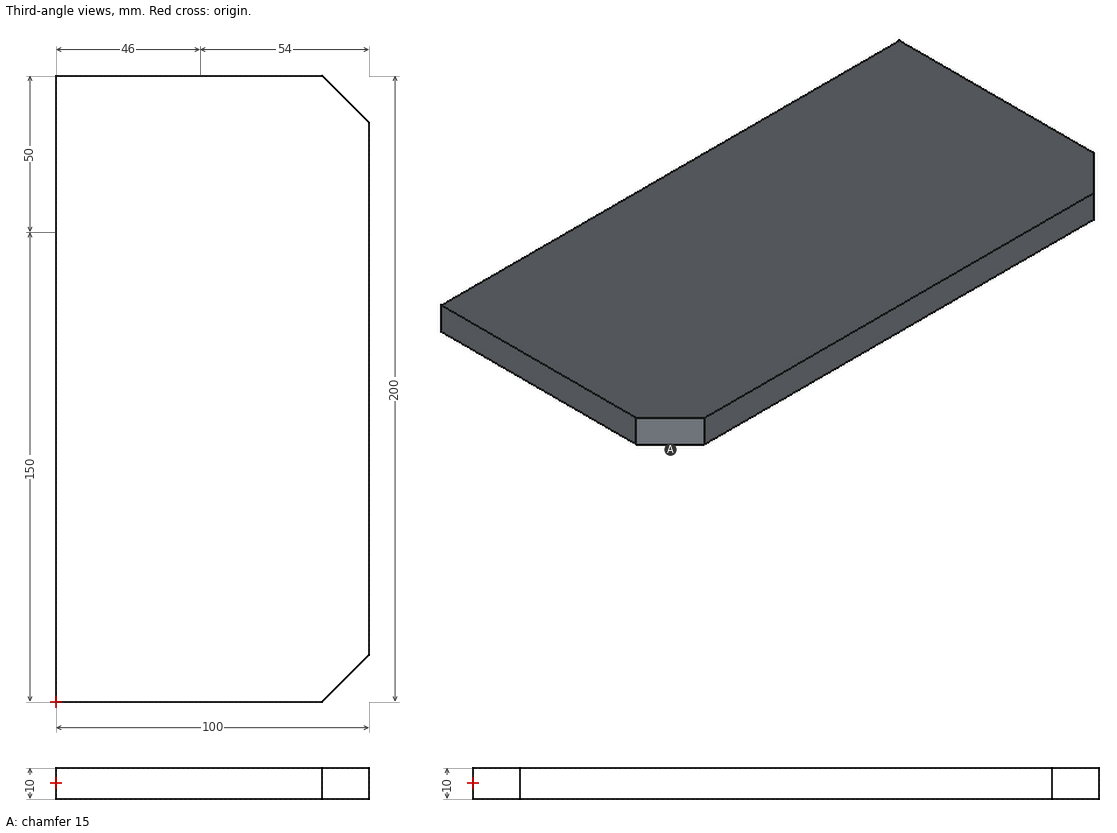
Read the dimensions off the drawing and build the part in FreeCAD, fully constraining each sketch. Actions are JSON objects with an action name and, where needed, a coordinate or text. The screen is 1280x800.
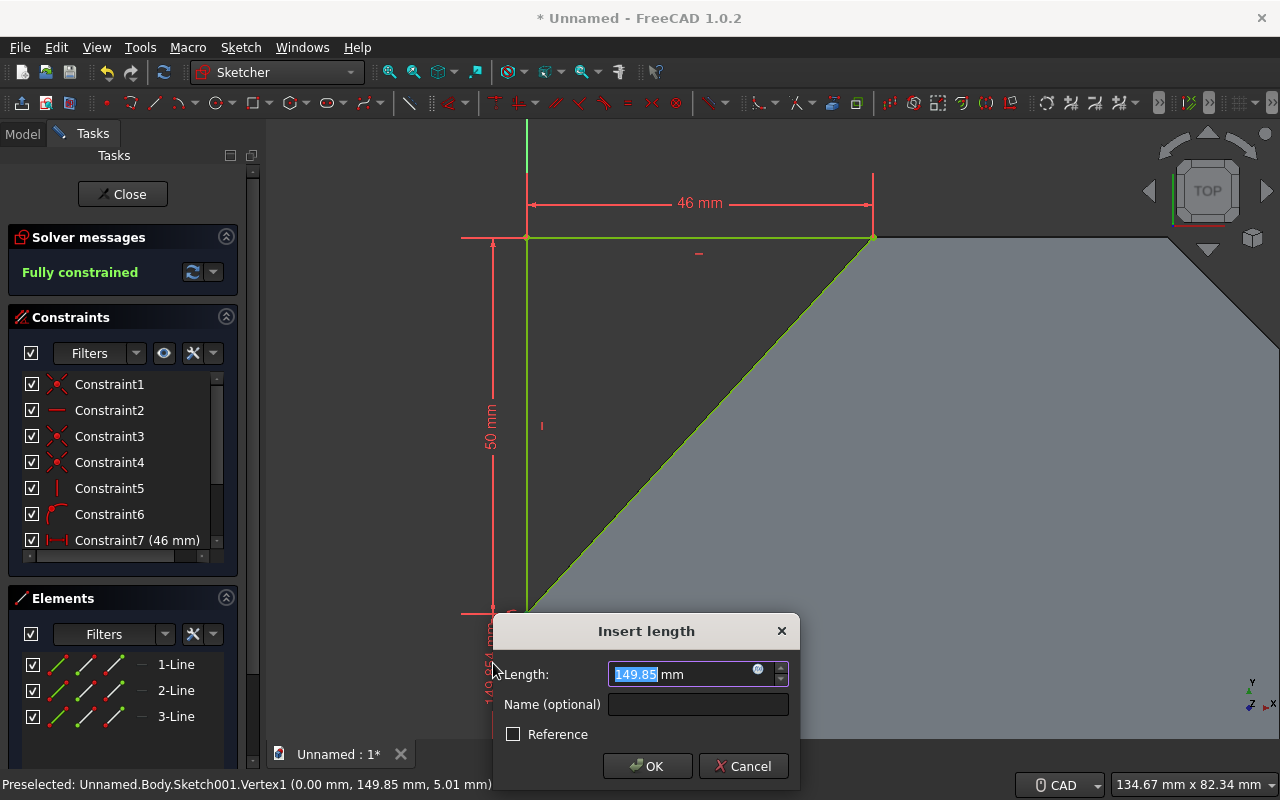
{"action": "type", "text": "150"}
{"action": "key", "text": "Return"}
{"action": "key", "text": "Escape"}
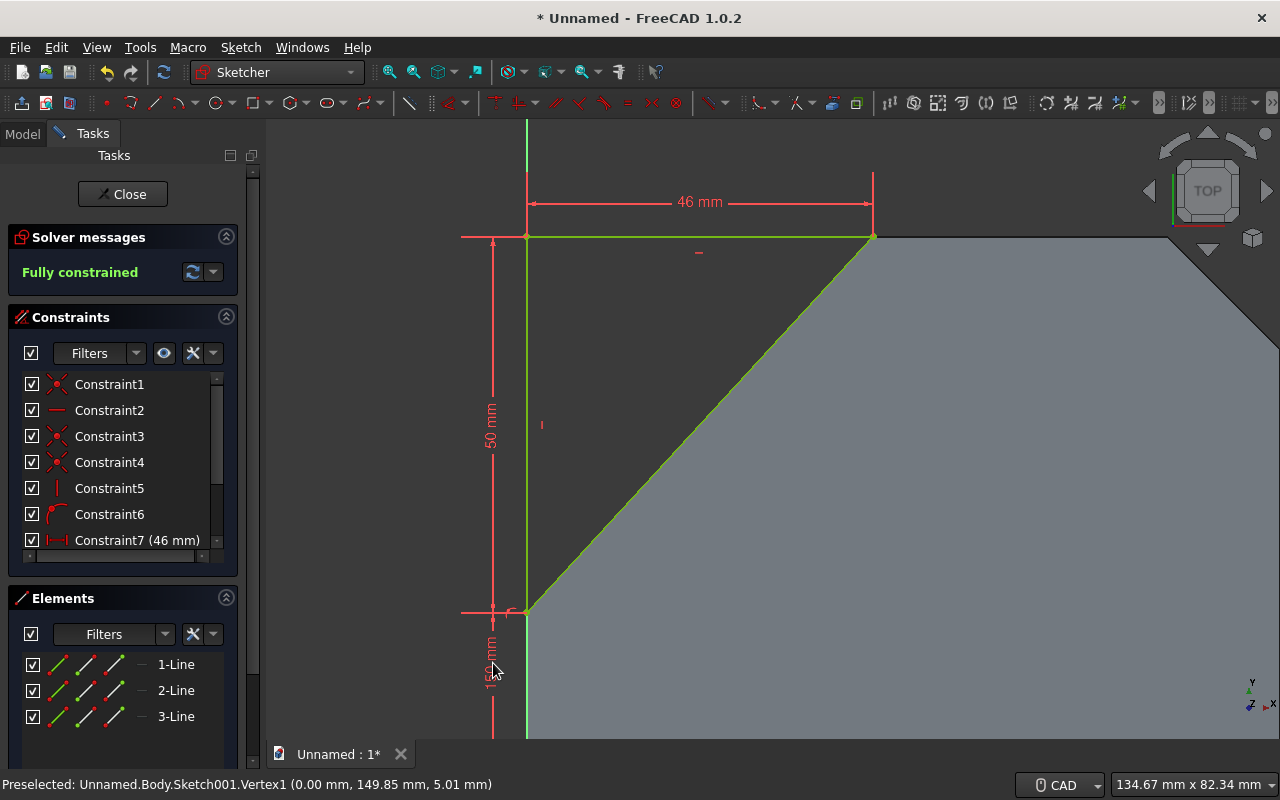
{"action": "left_click", "coordinate": [123, 194]}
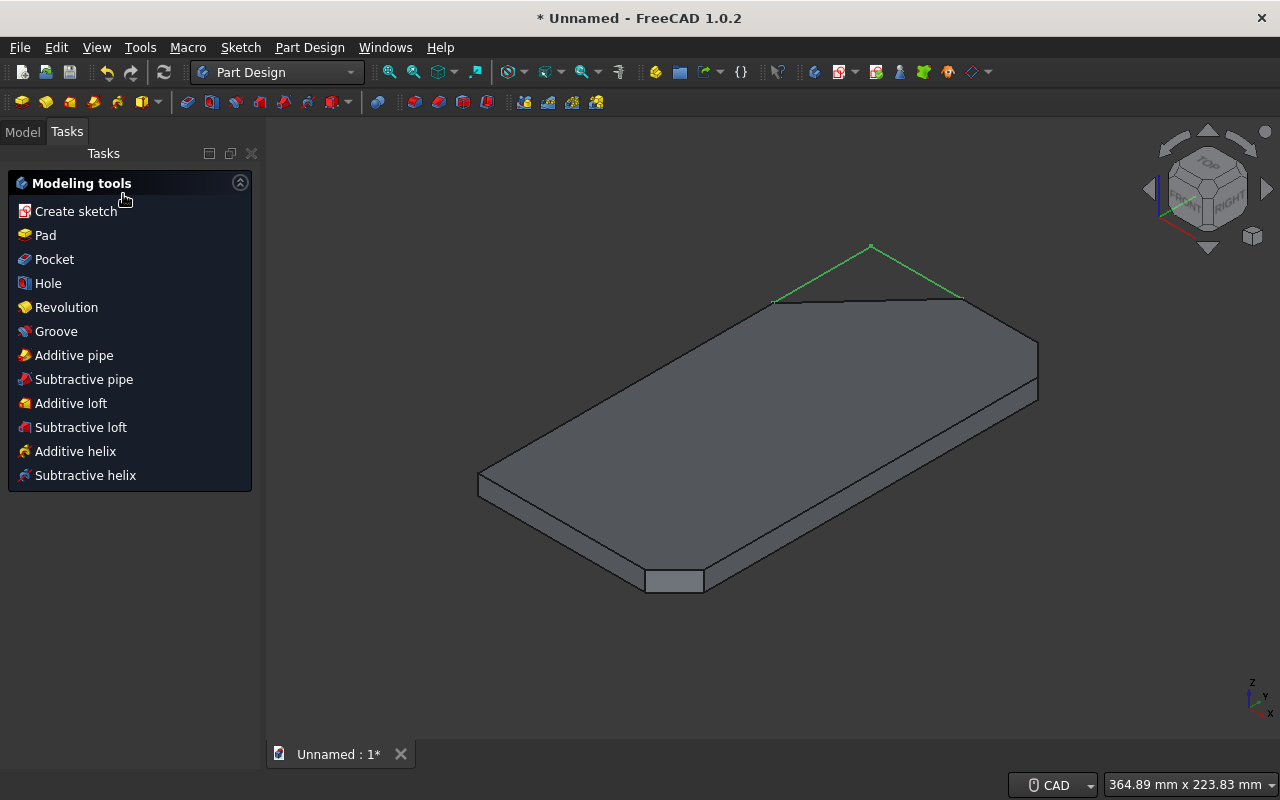
{"action": "left_click", "coordinate": [22, 102]}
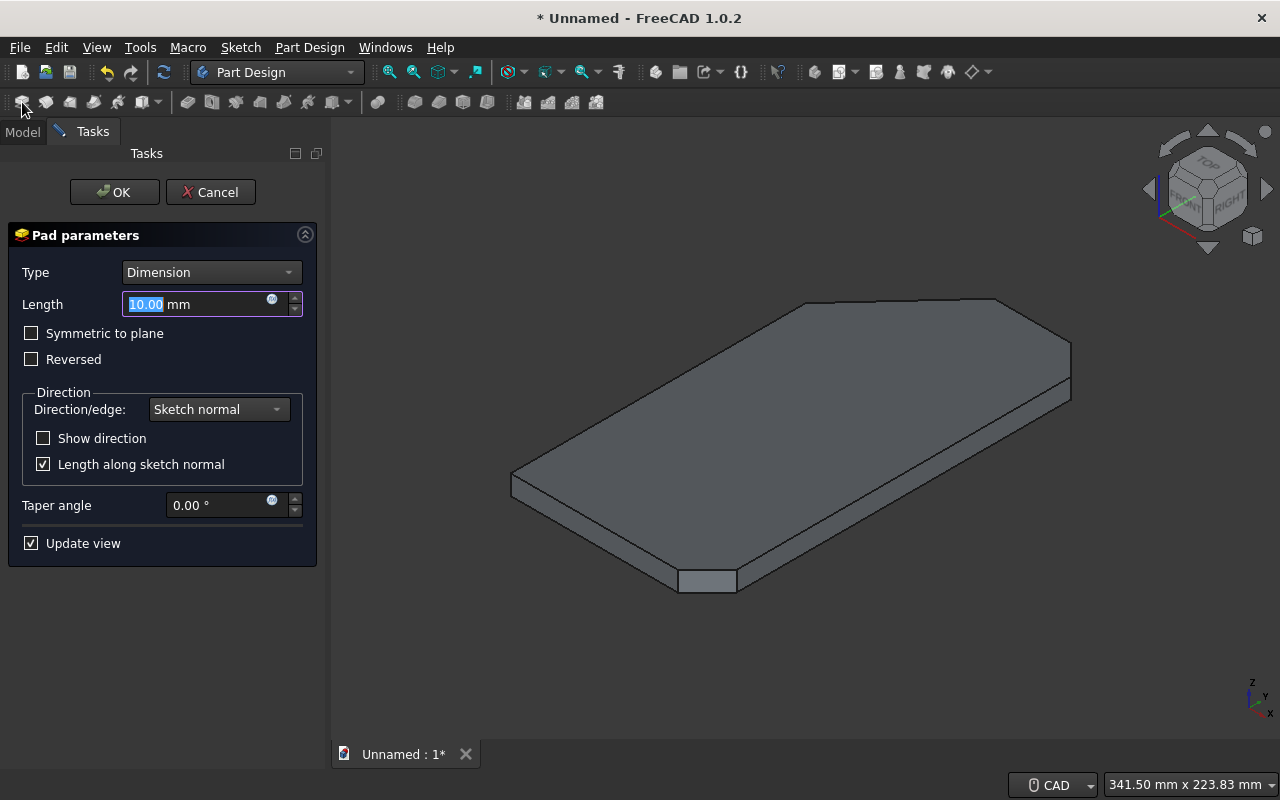
{"action": "type", "text": "10"}
{"action": "key", "text": "Tab"}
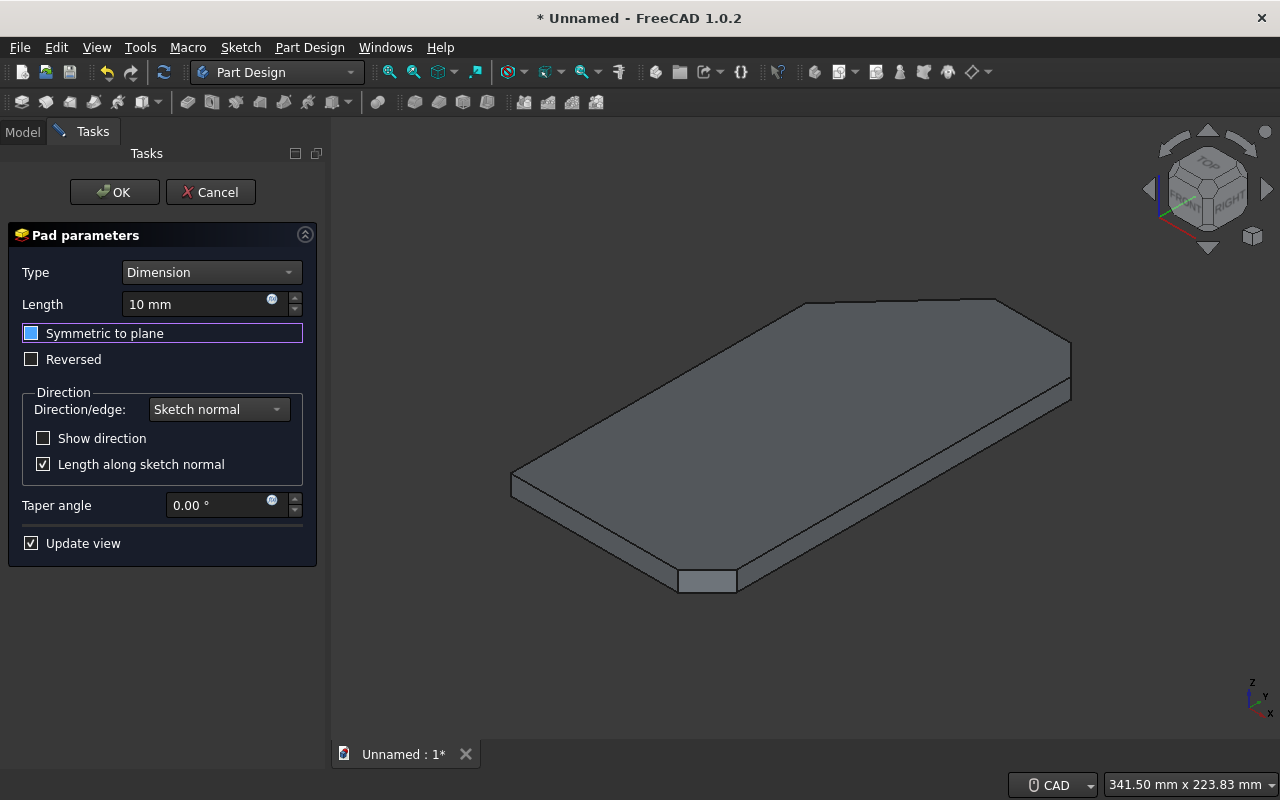
{"action": "left_click", "coordinate": [30, 359]}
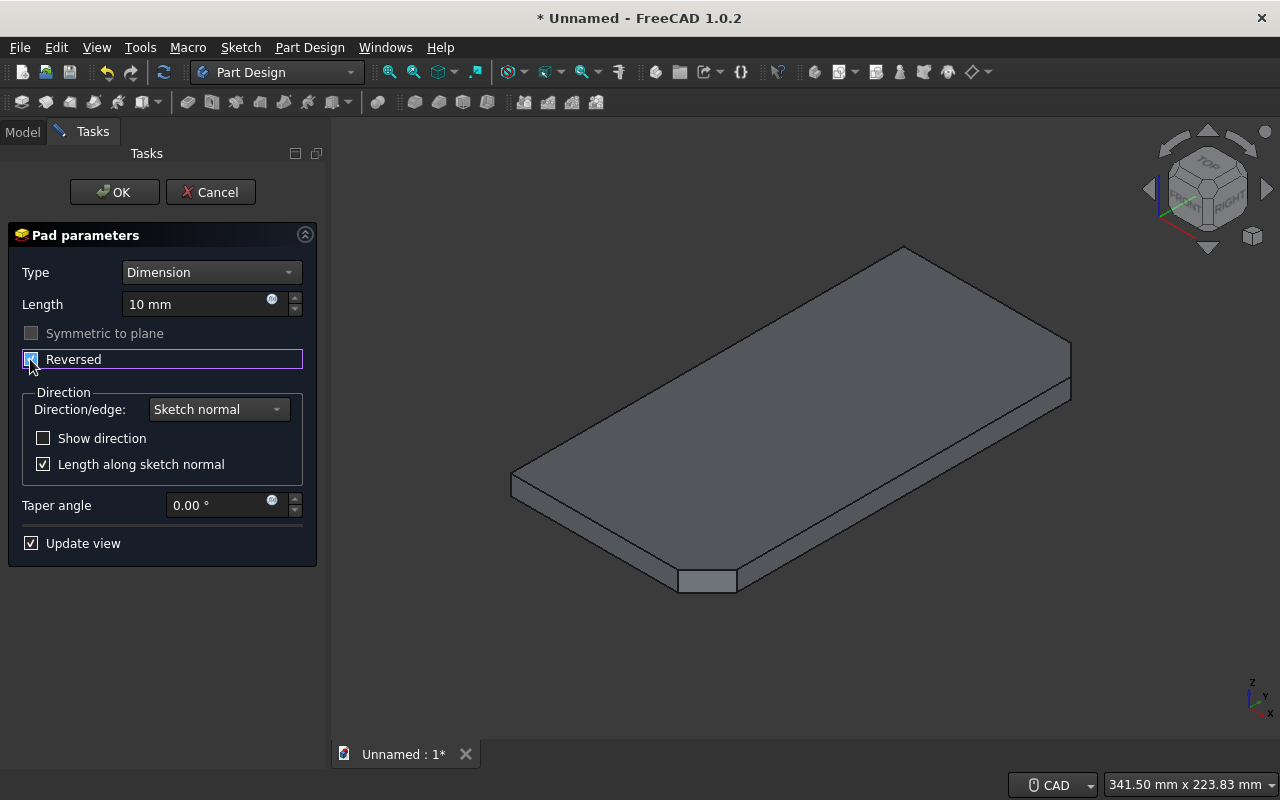
{"action": "left_click", "coordinate": [115, 192]}